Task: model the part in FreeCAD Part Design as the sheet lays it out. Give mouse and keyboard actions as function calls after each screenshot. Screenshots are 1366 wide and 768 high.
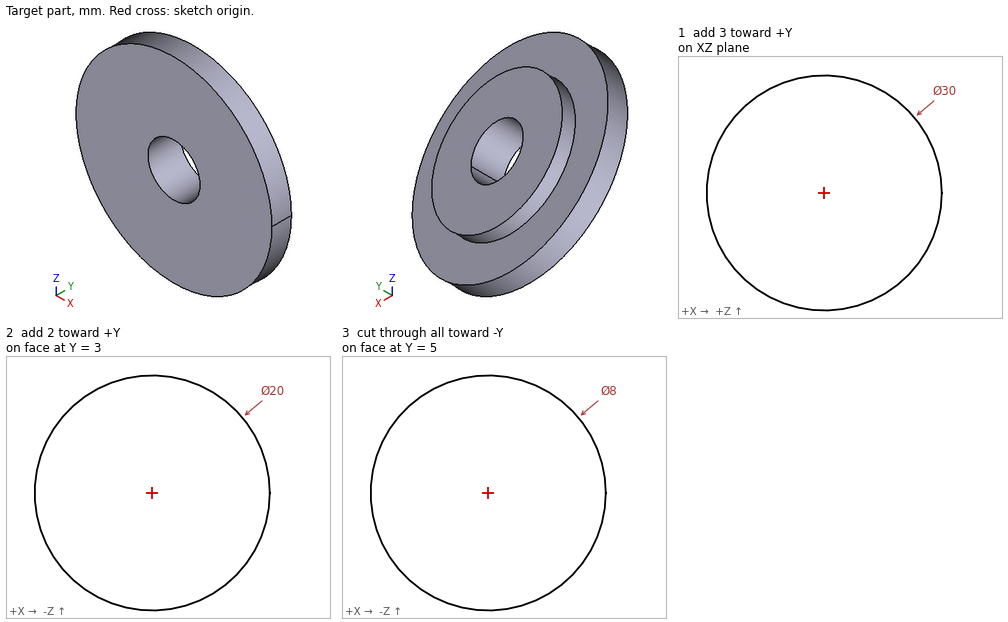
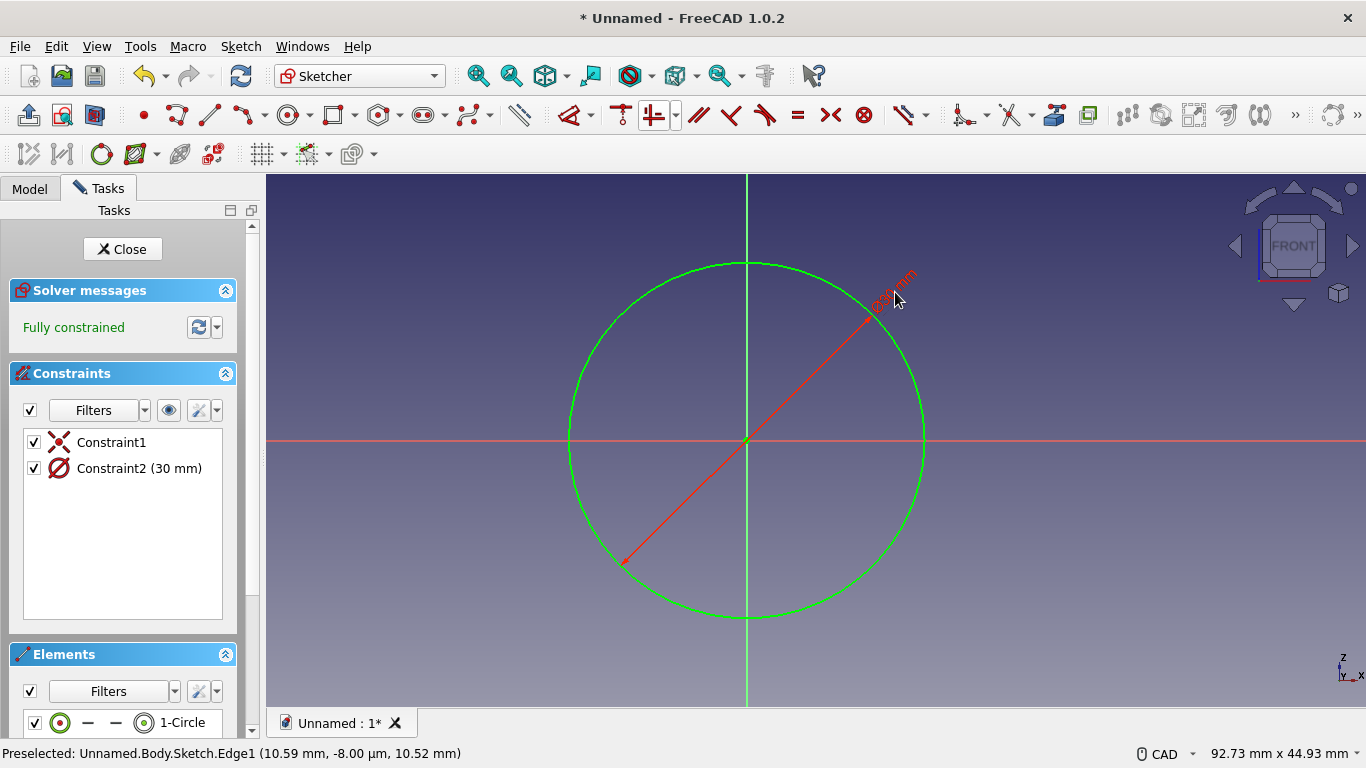
click(123, 249)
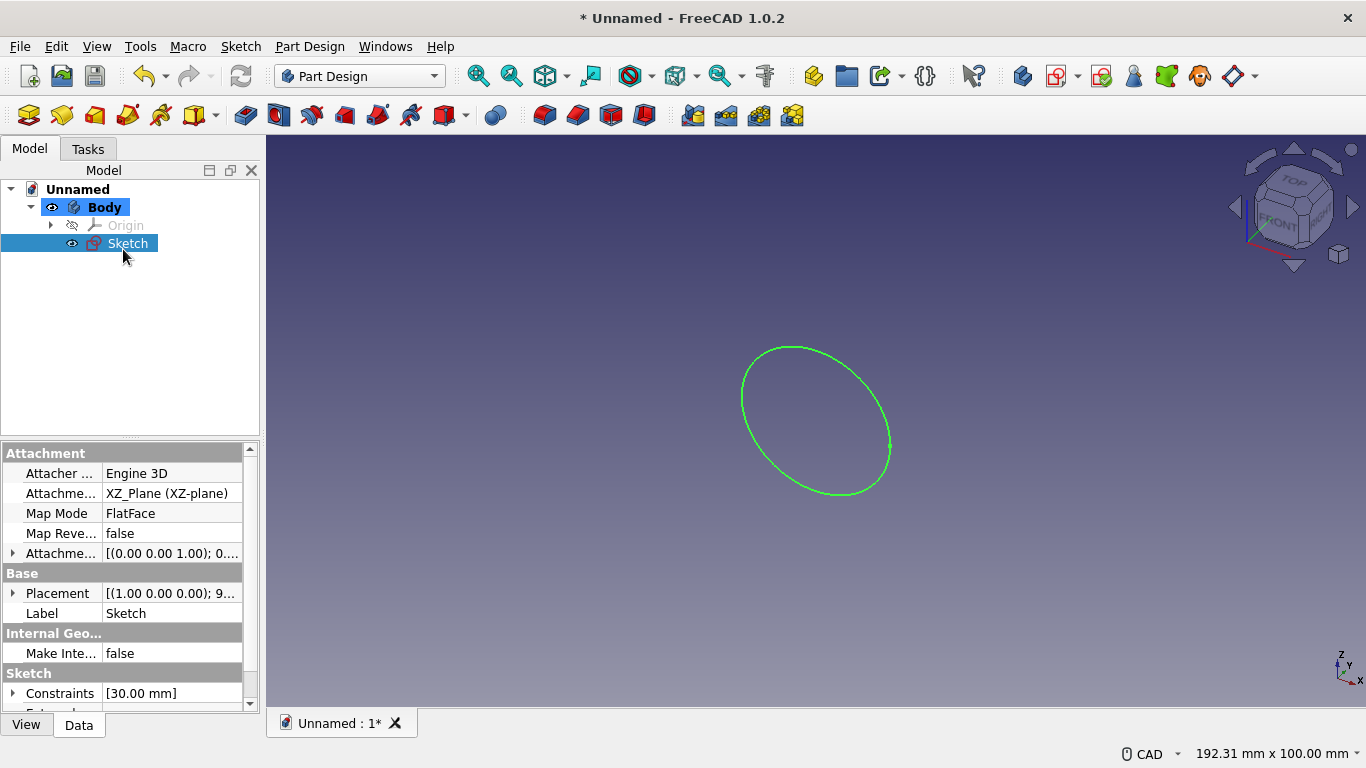
click(29, 116)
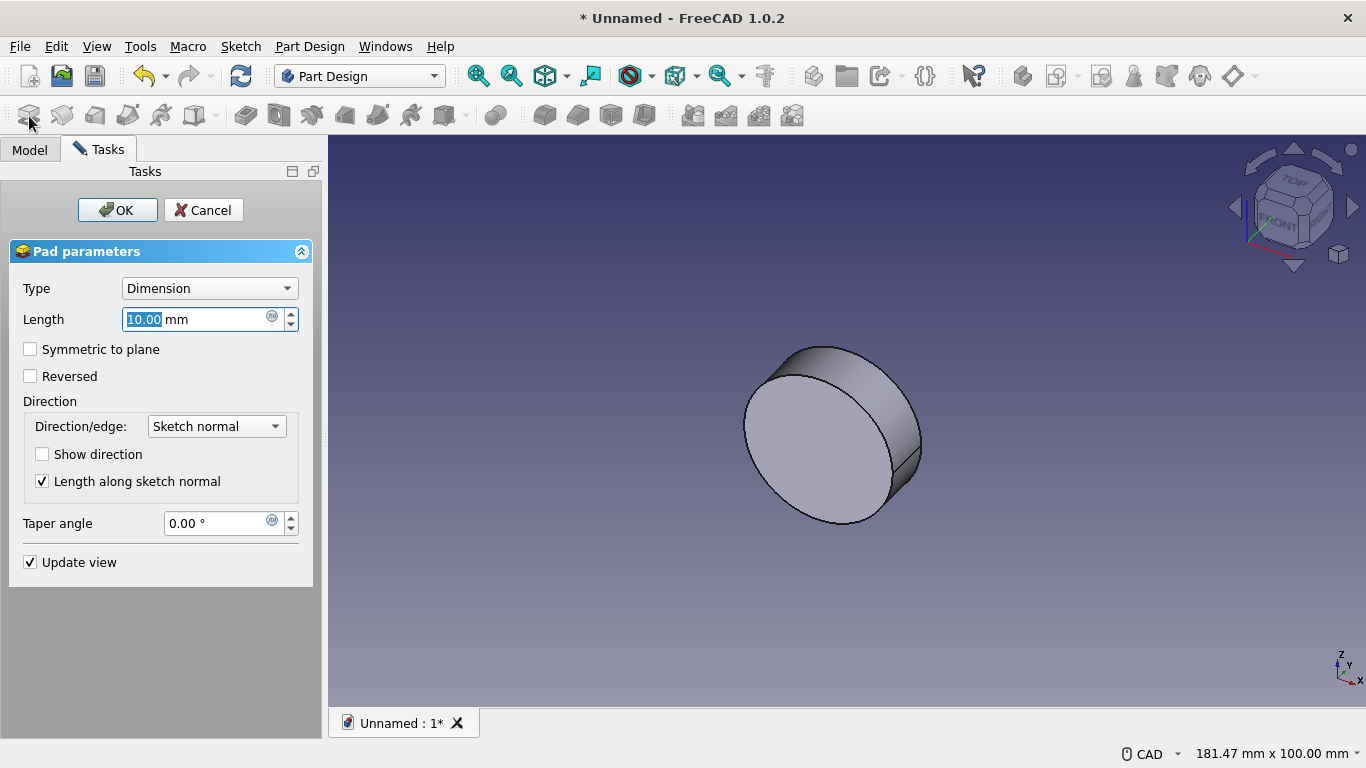
text(3)
key(Tab)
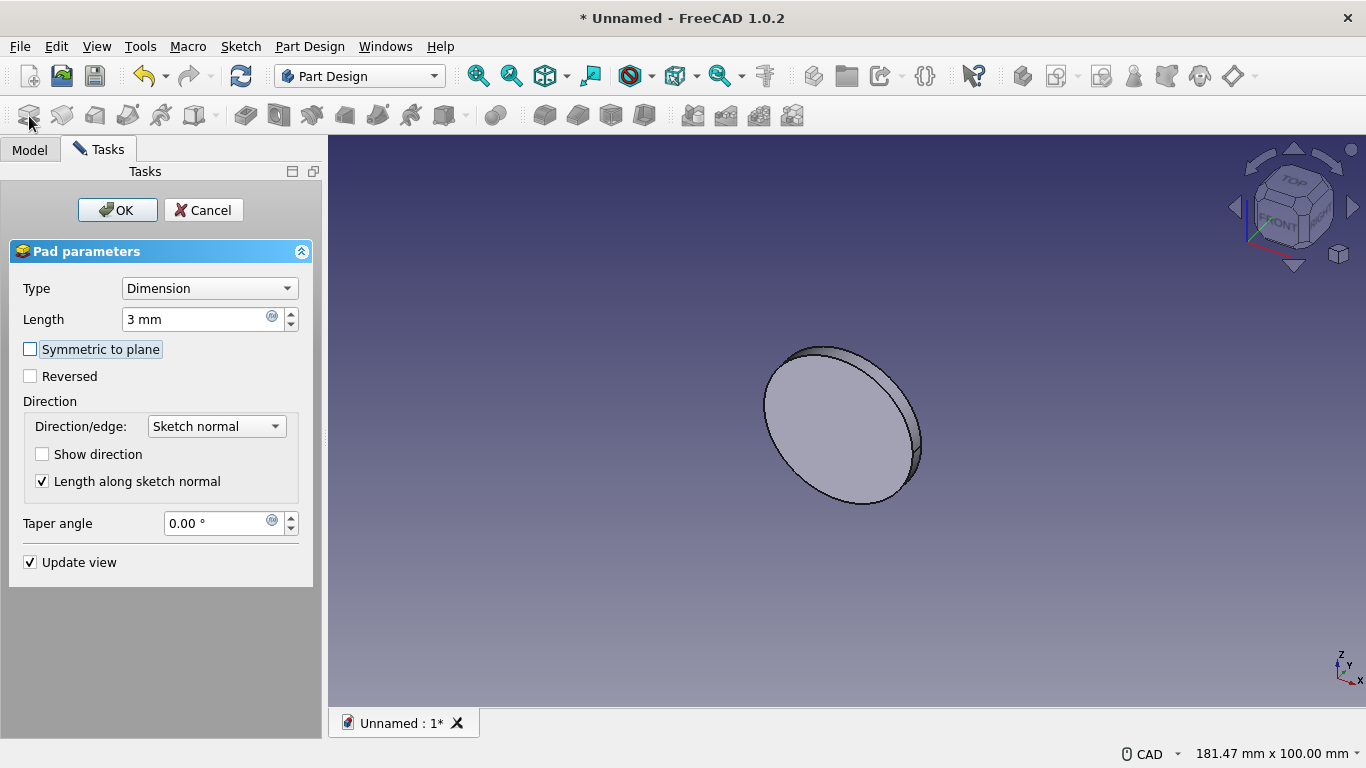
click(31, 376)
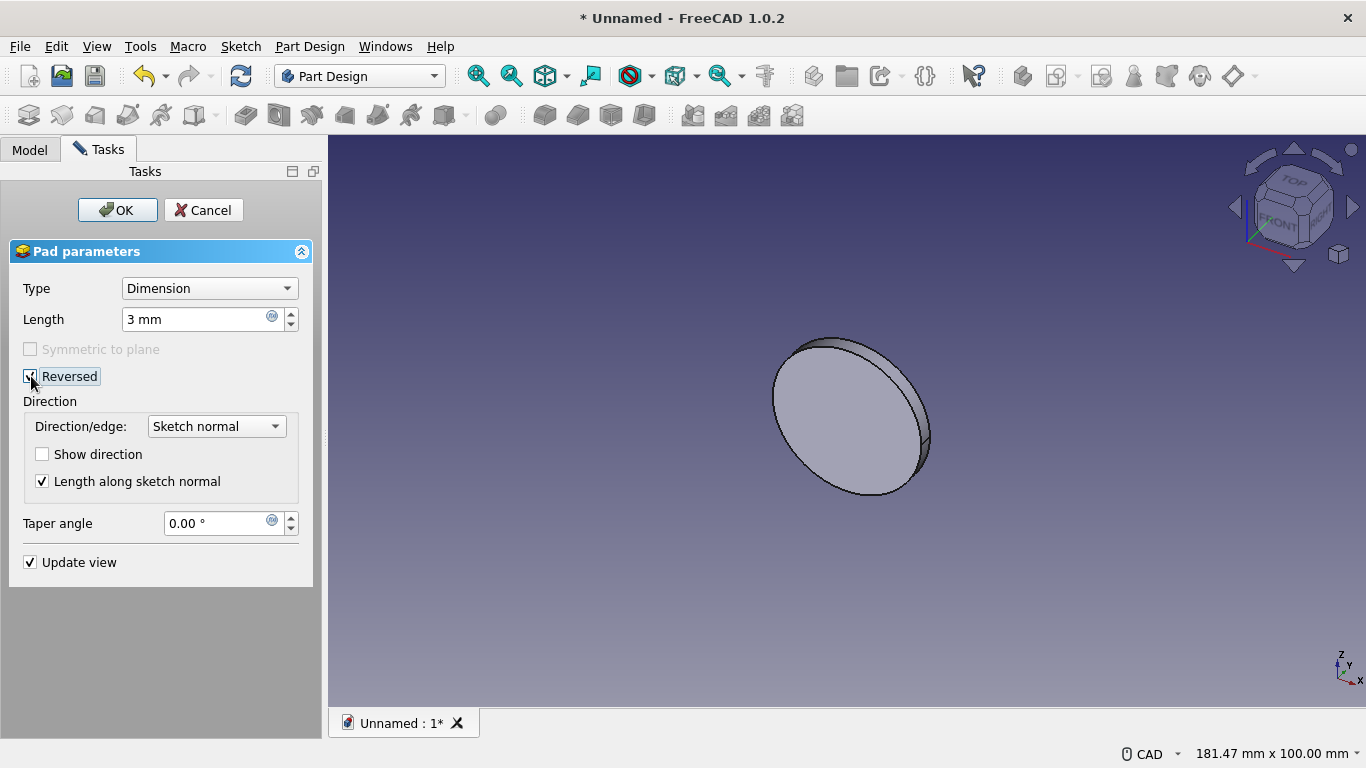
click(118, 210)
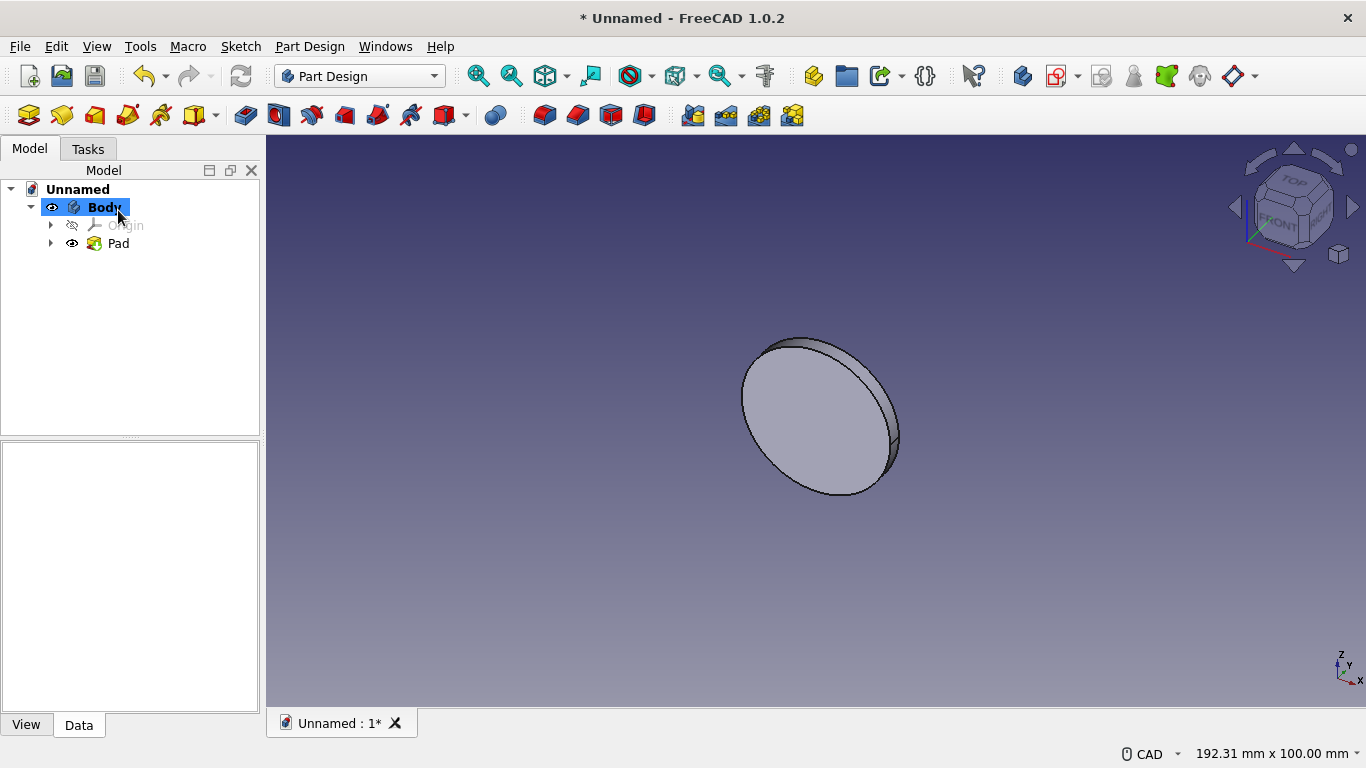
click(479, 76)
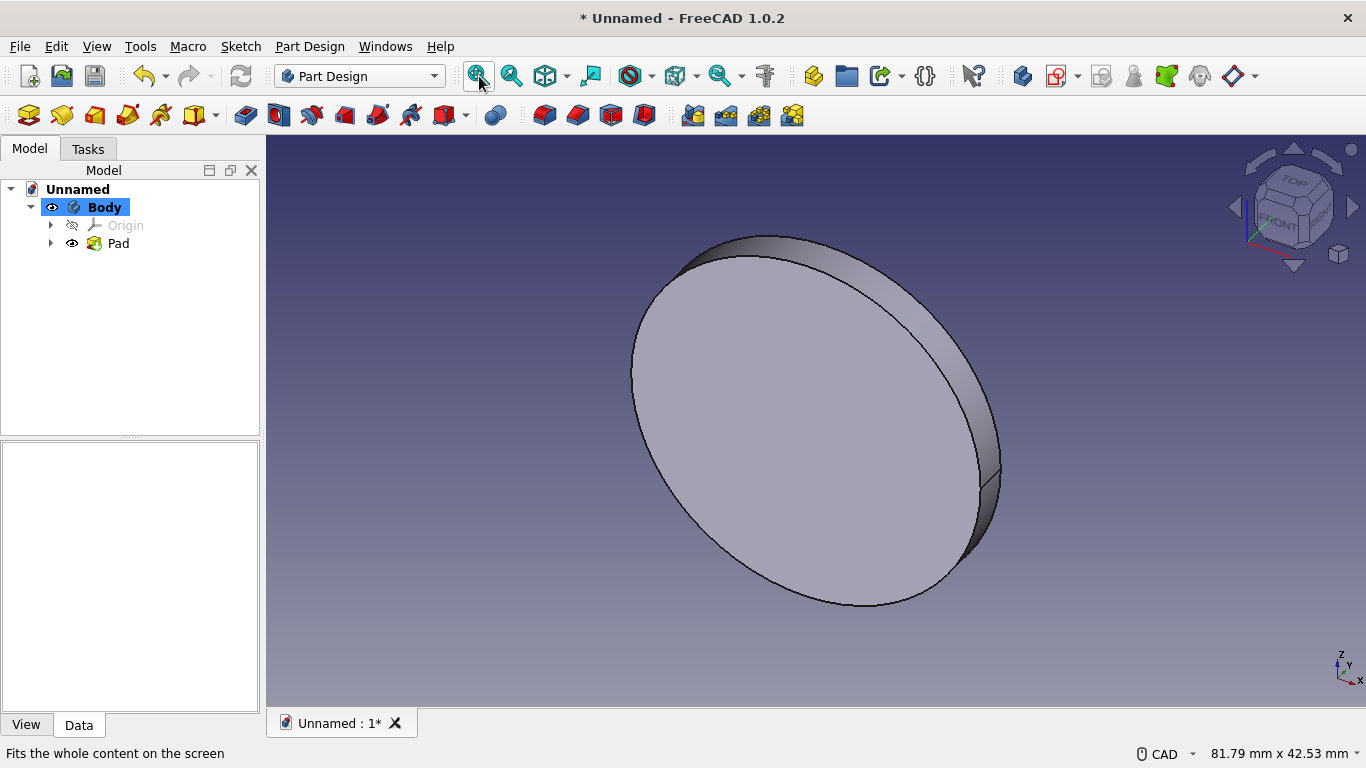
key(4)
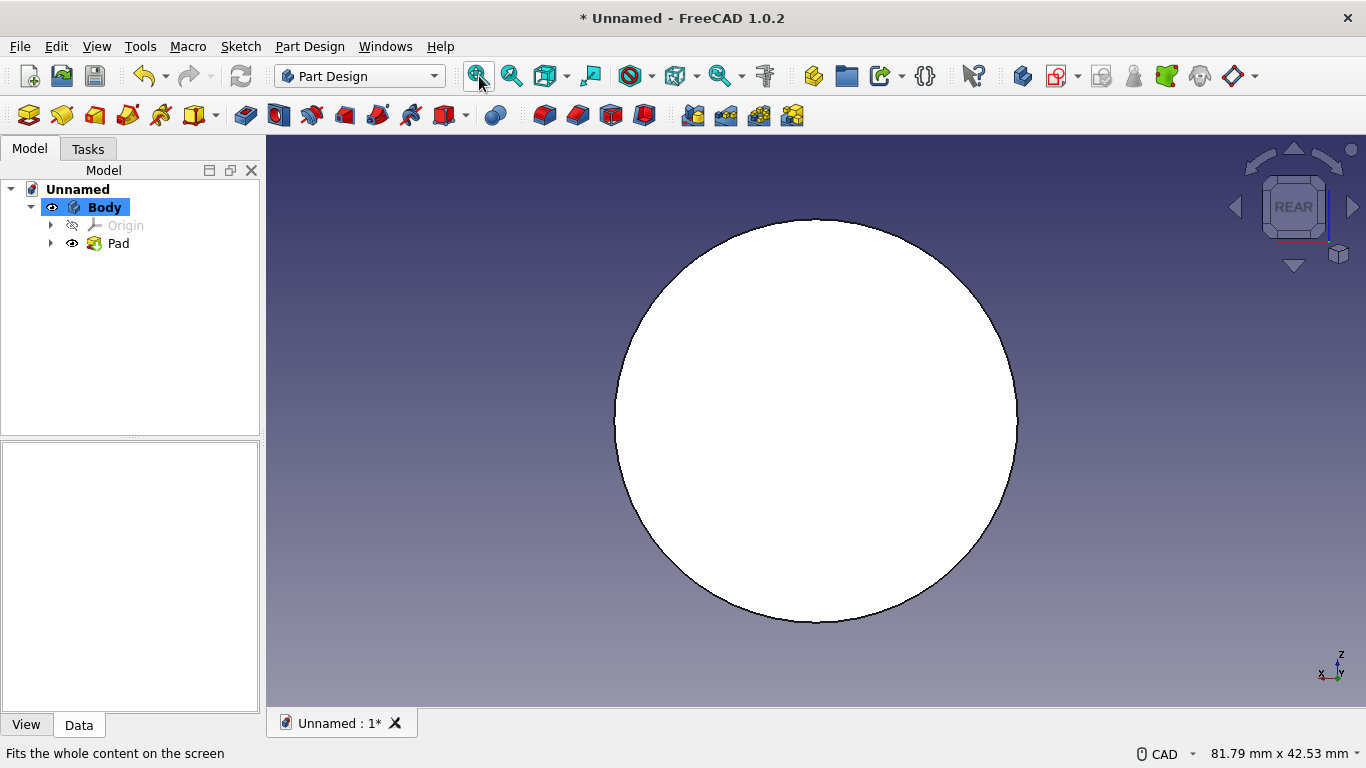
click(816, 420)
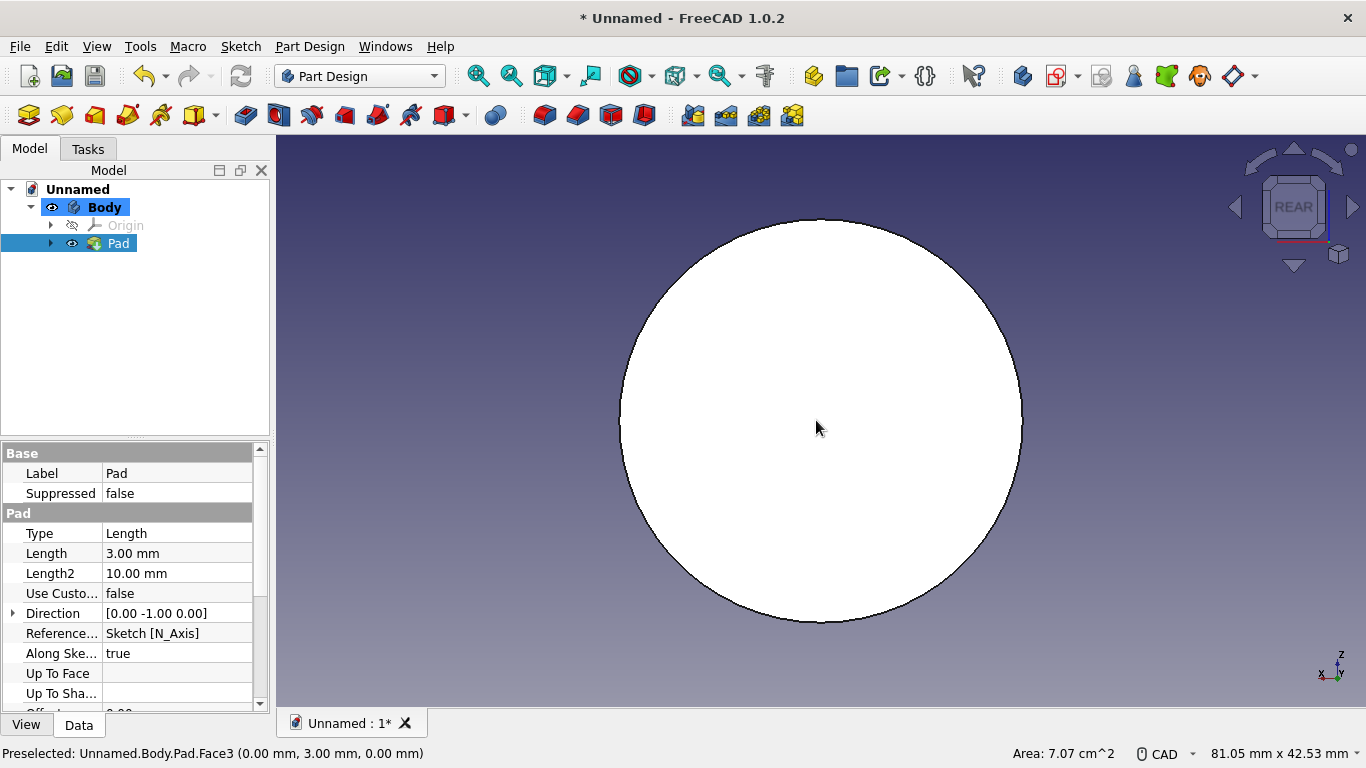
click(1056, 76)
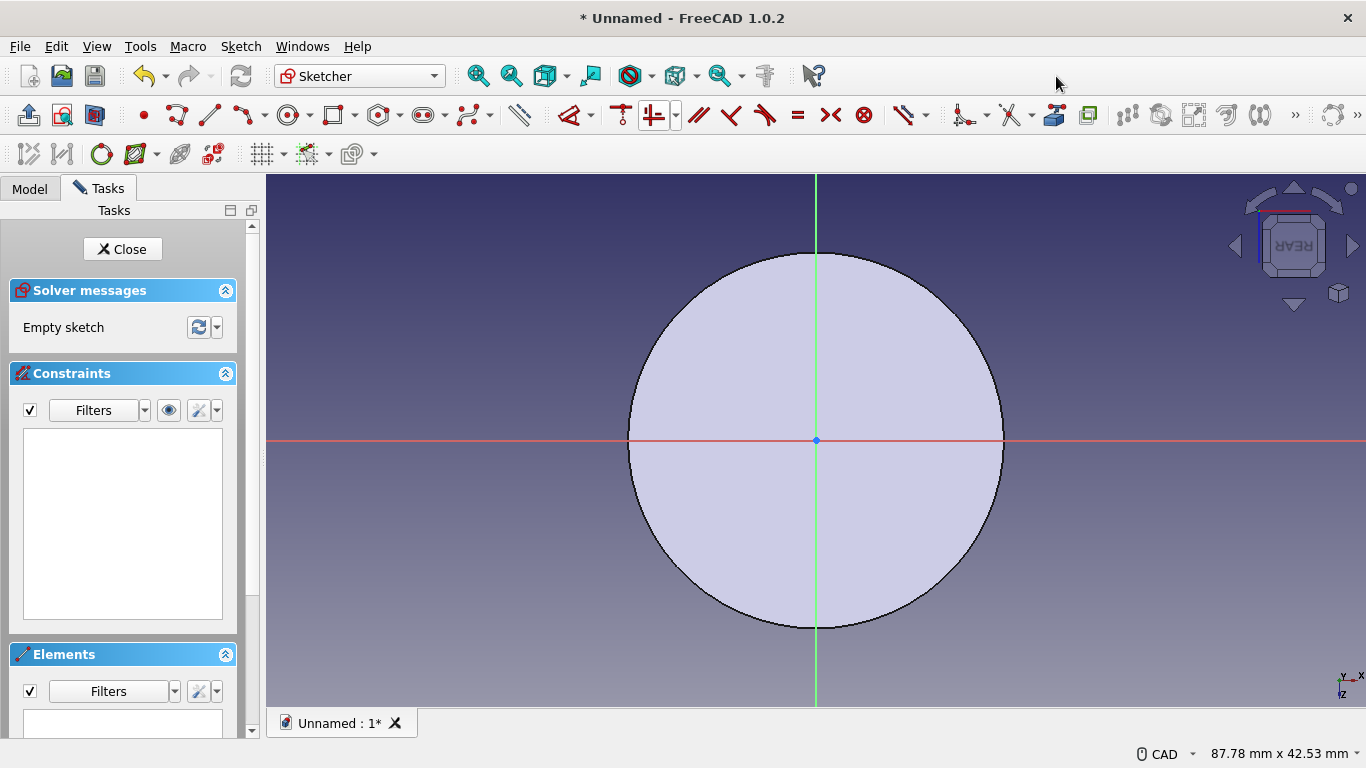
click(288, 116)